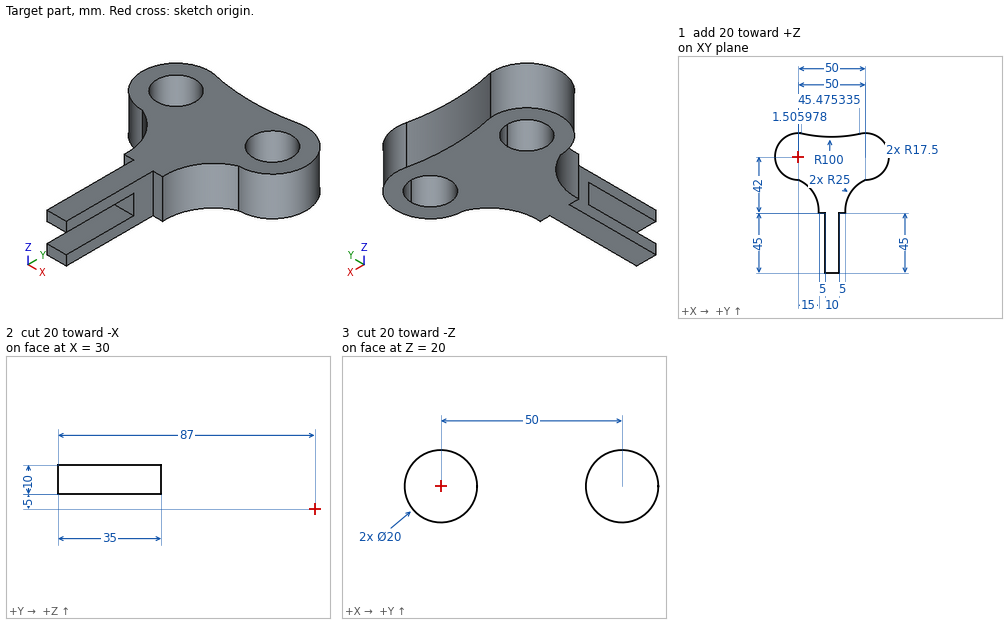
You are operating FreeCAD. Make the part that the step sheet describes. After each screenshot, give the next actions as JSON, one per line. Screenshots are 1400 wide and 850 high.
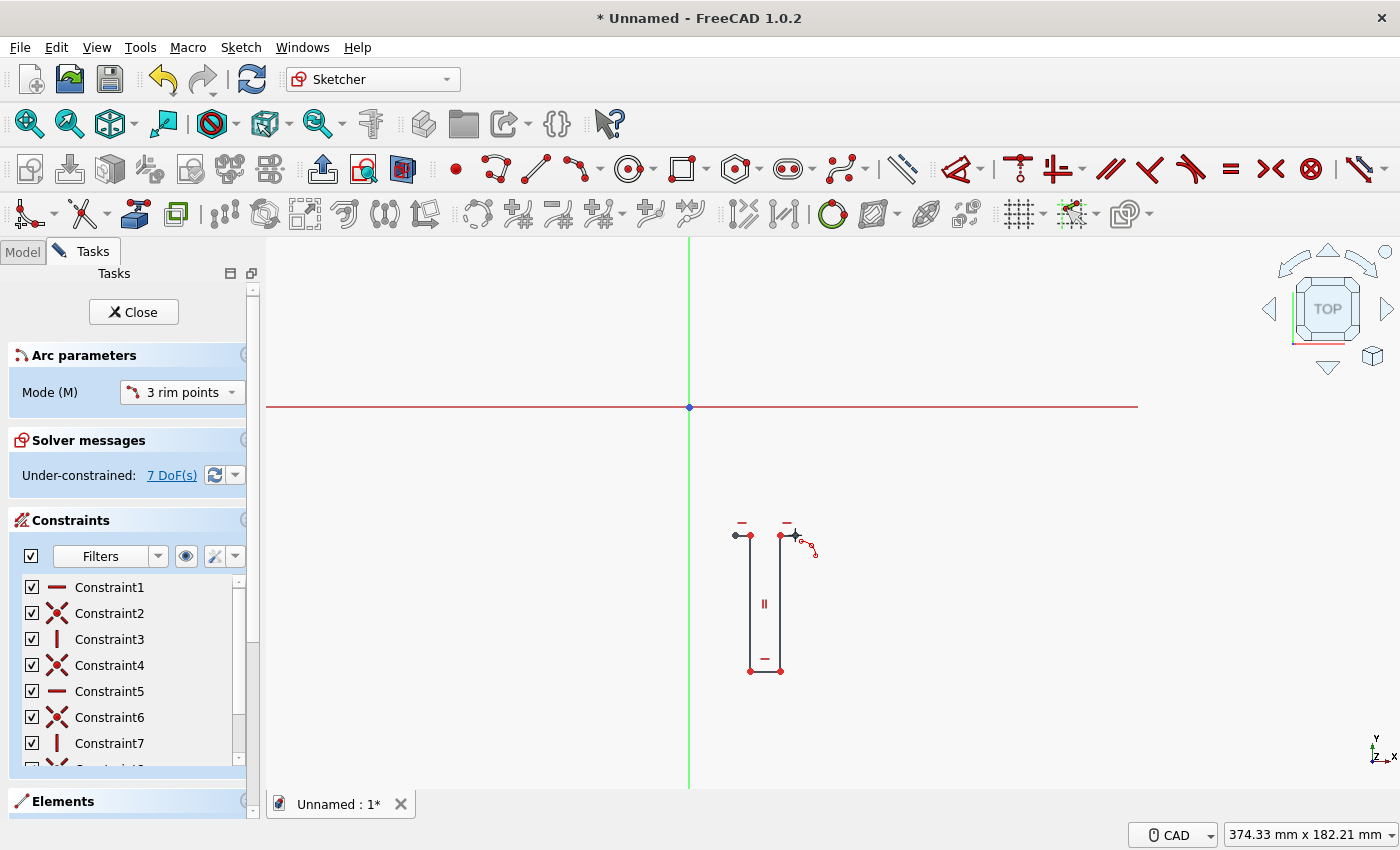
{"action": "scroll", "coordinate": [795, 535], "scroll_direction": "up", "scroll_amount": 4}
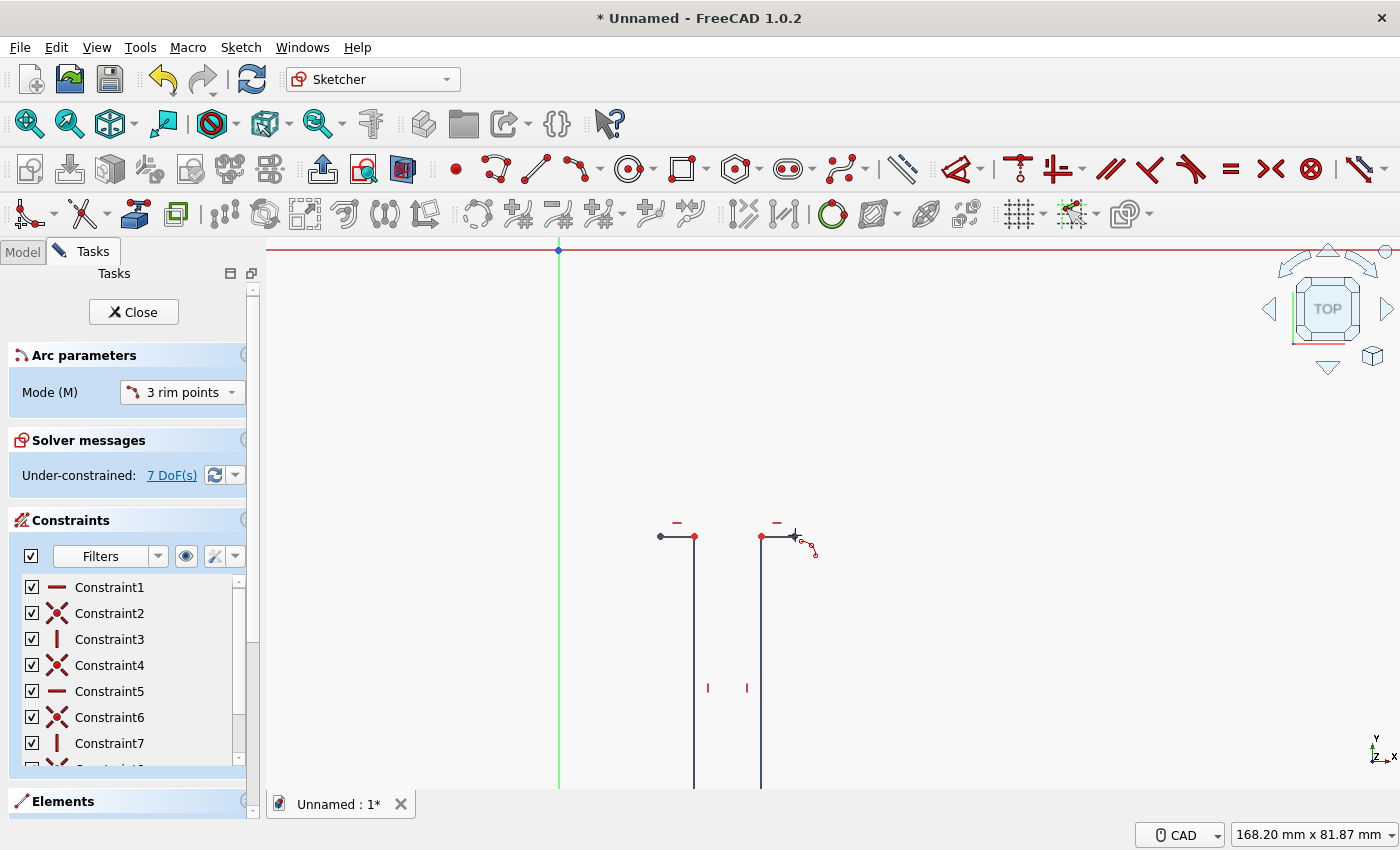
{"action": "left_click", "coordinate": [794, 537]}
{"action": "left_click", "coordinate": [896, 368]}
{"action": "left_click", "coordinate": [819, 435]}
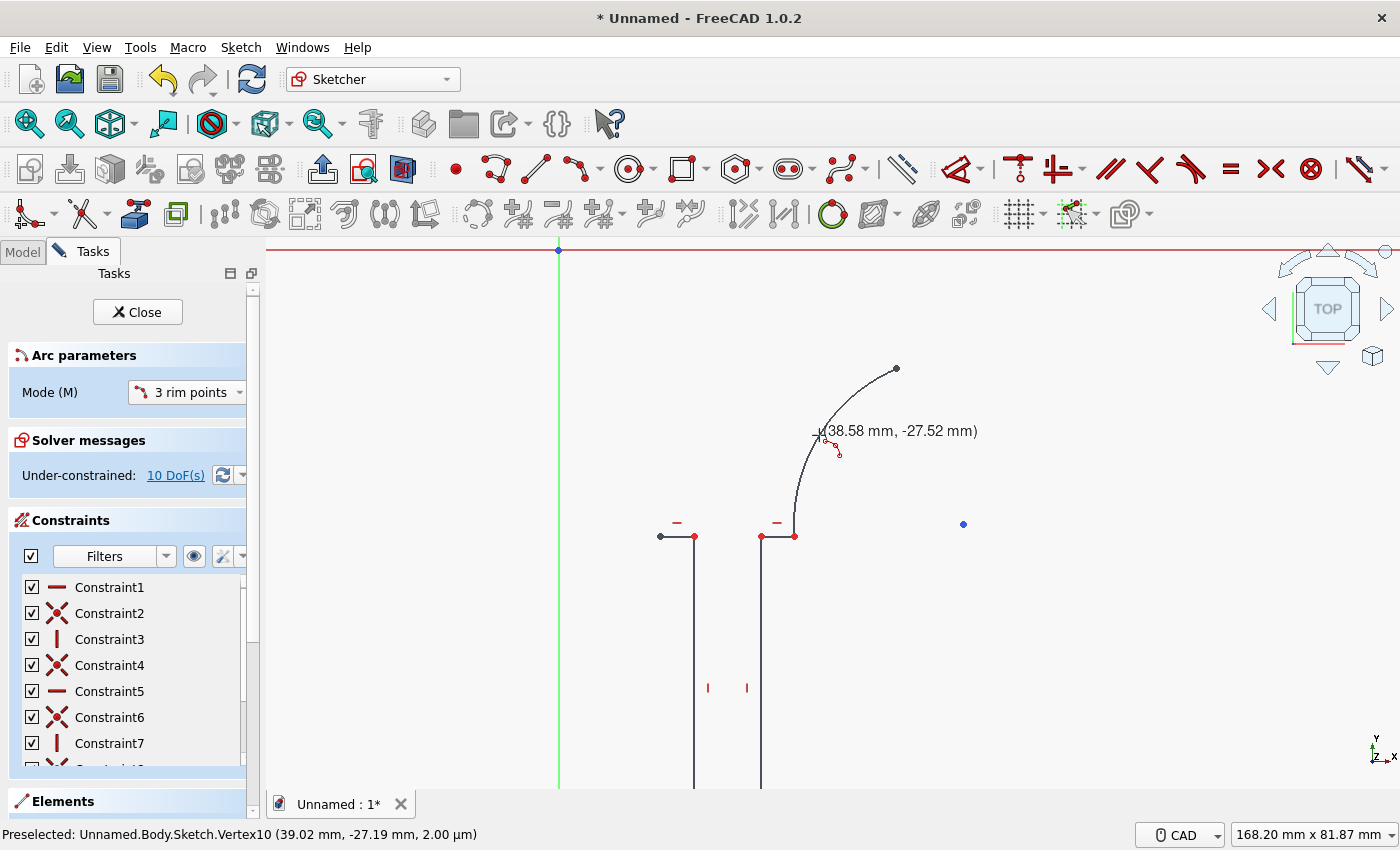
{"action": "left_click", "coordinate": [896, 369]}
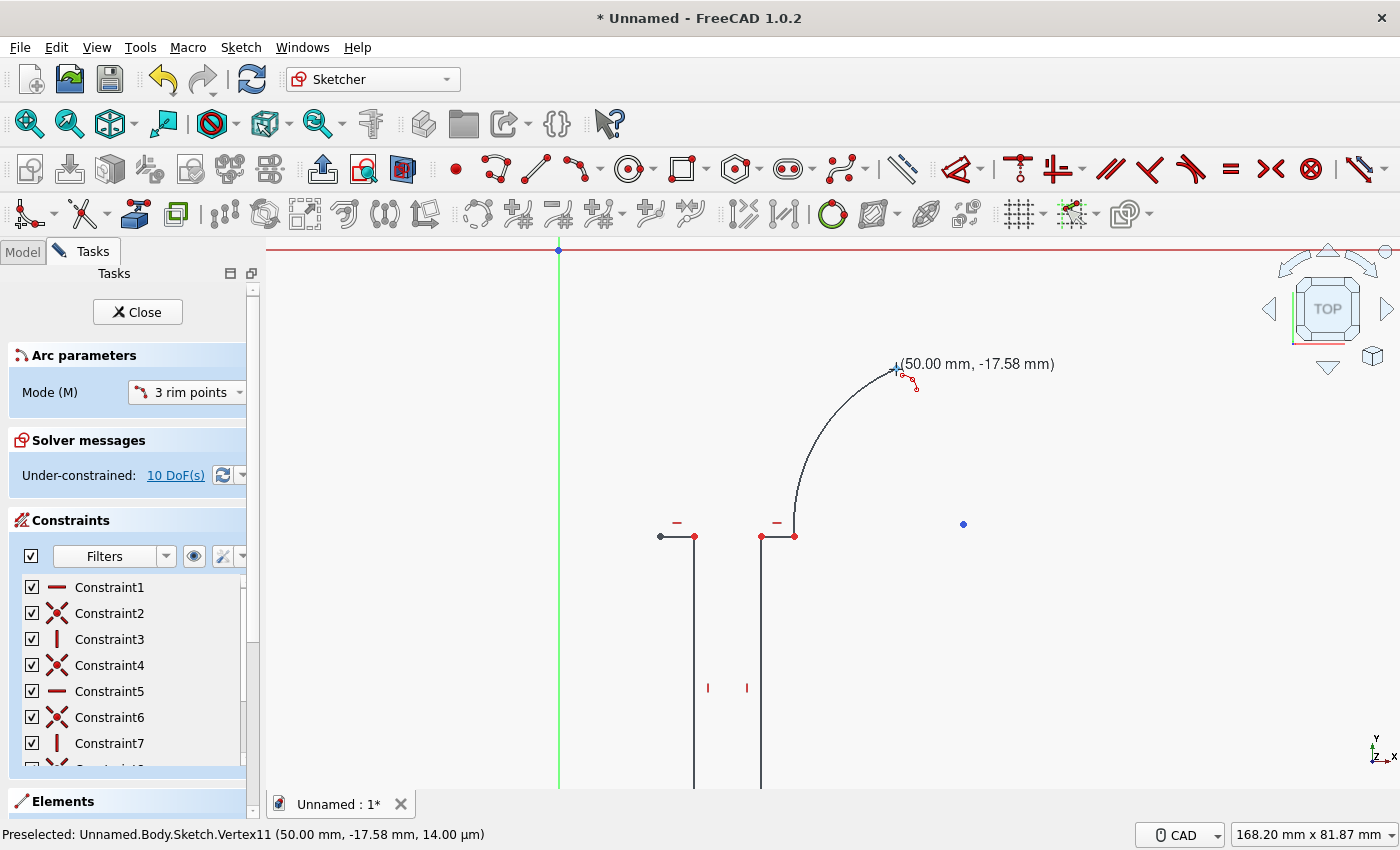
{"action": "scroll", "coordinate": [810, 547], "scroll_direction": "down", "scroll_amount": 3}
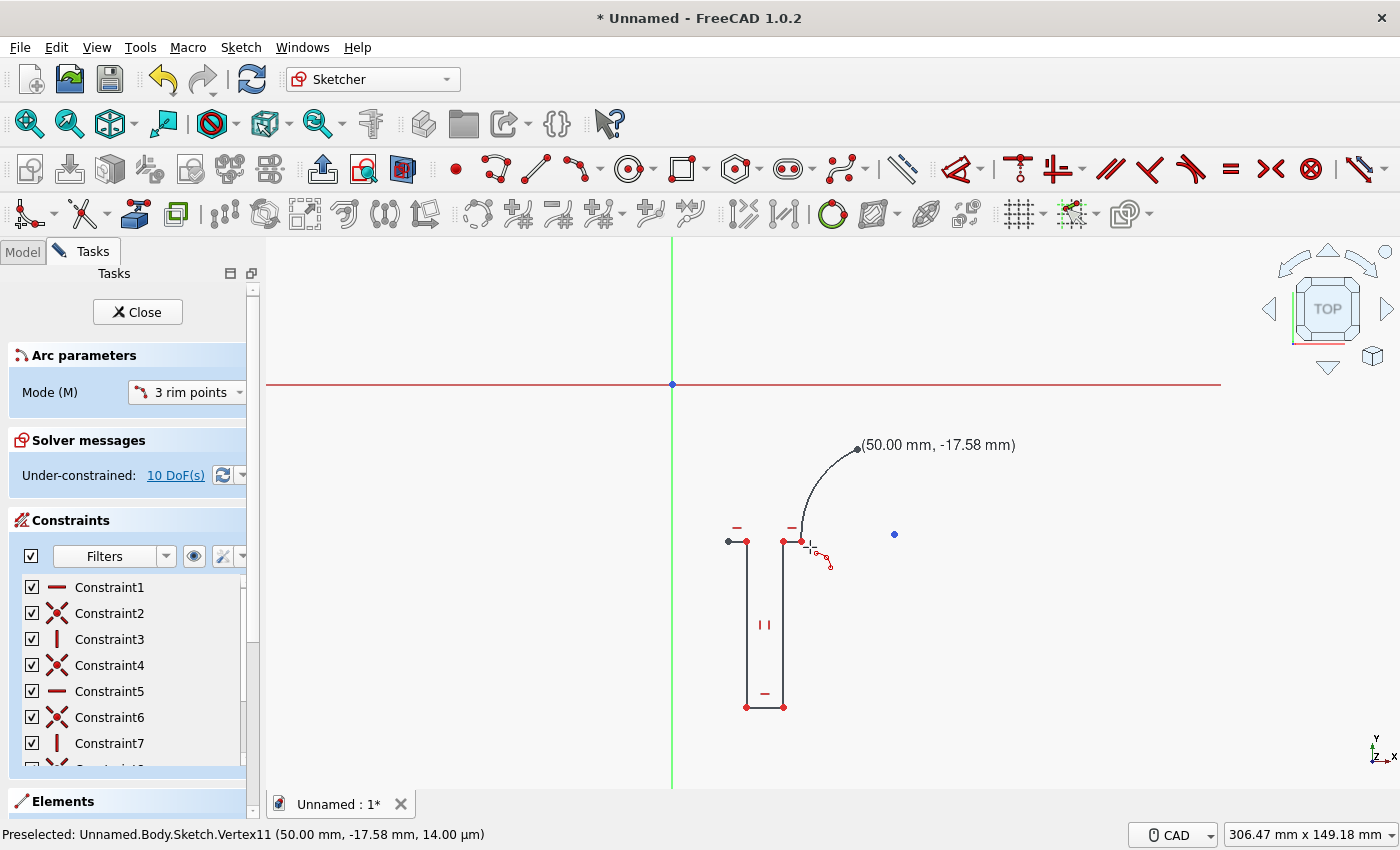
{"action": "left_click", "coordinate": [841, 322]}
{"action": "left_click", "coordinate": [915, 355]}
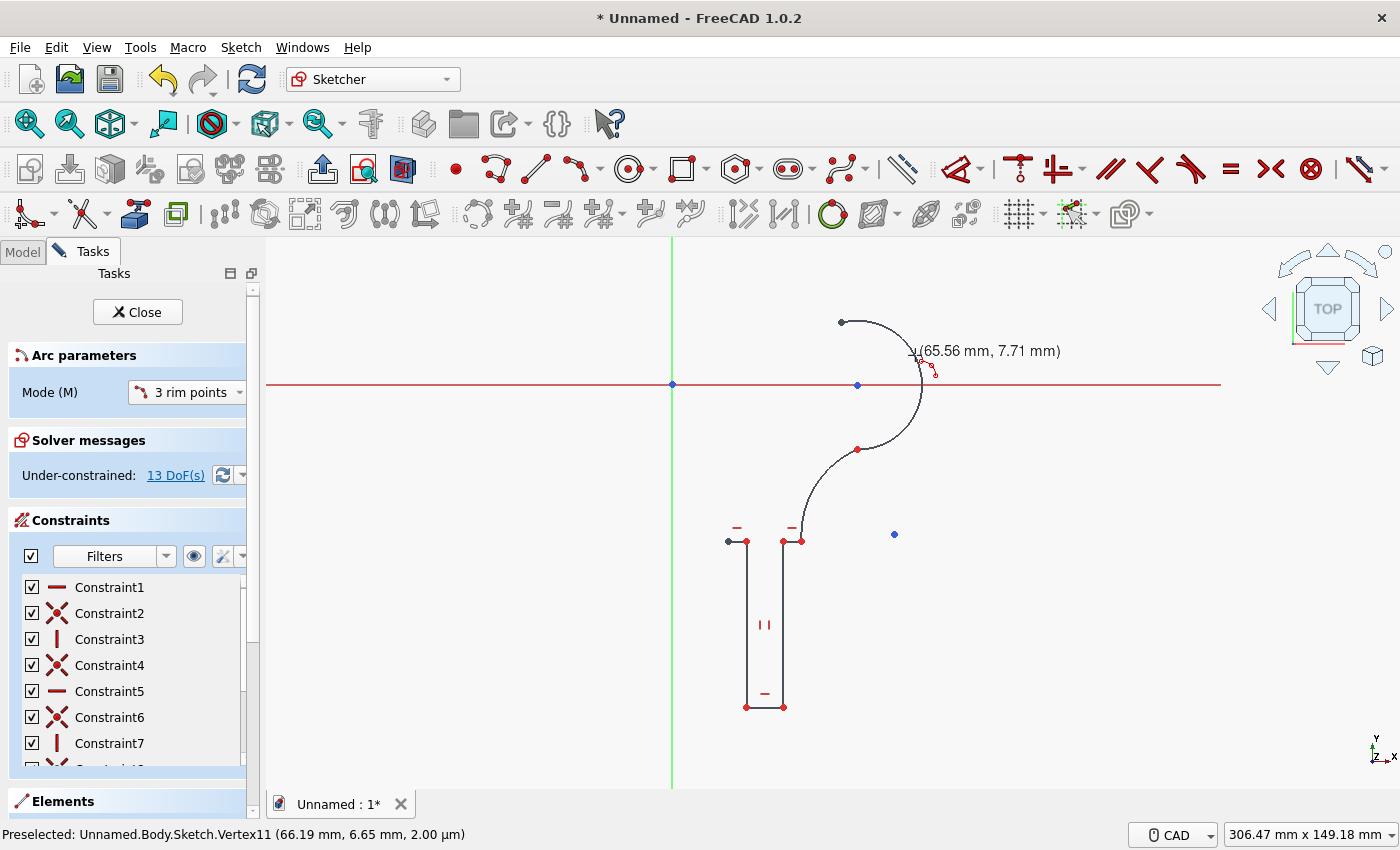
{"action": "left_click", "coordinate": [841, 323]}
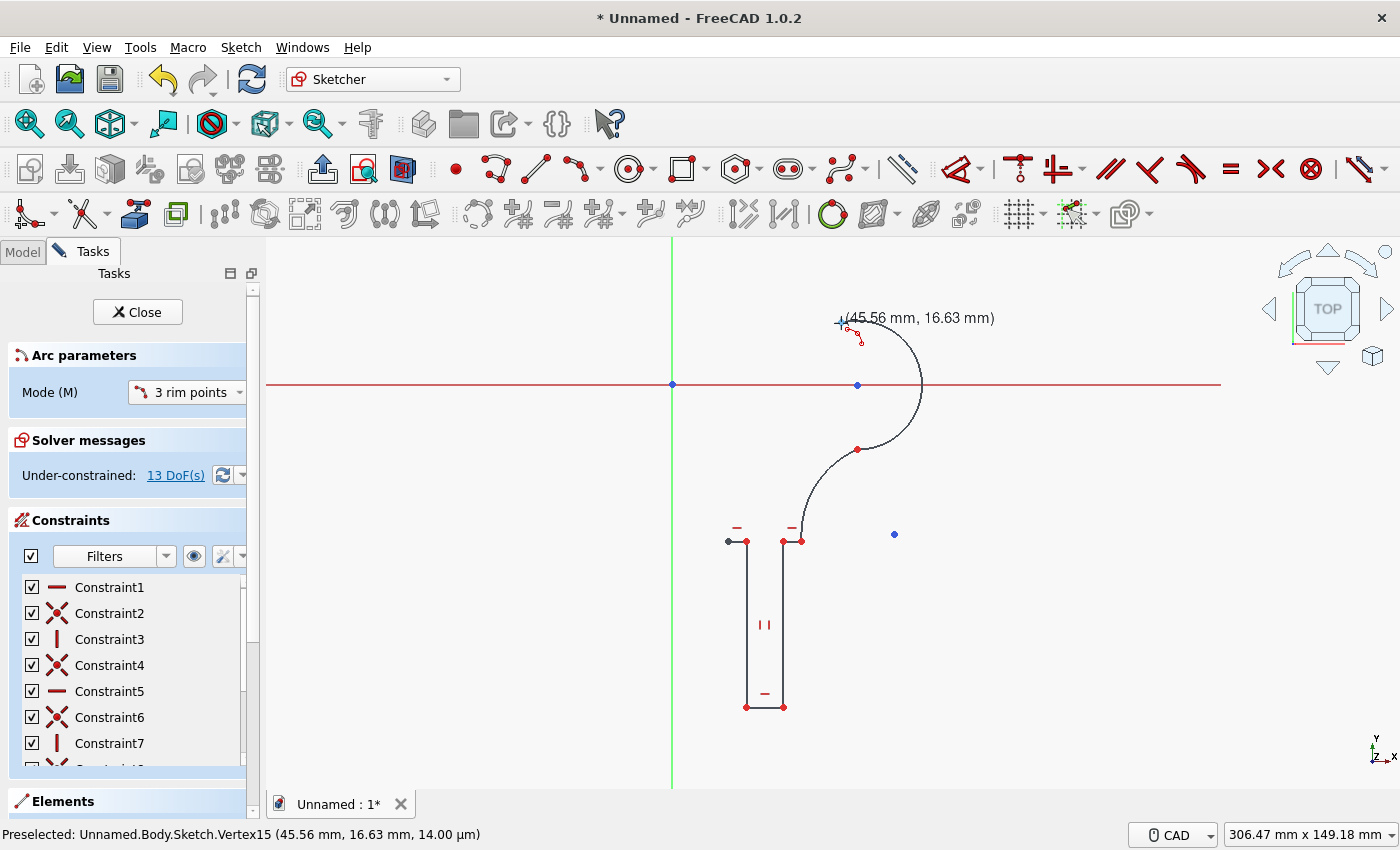
{"action": "scroll", "coordinate": [678, 320], "scroll_direction": "up", "scroll_amount": 6}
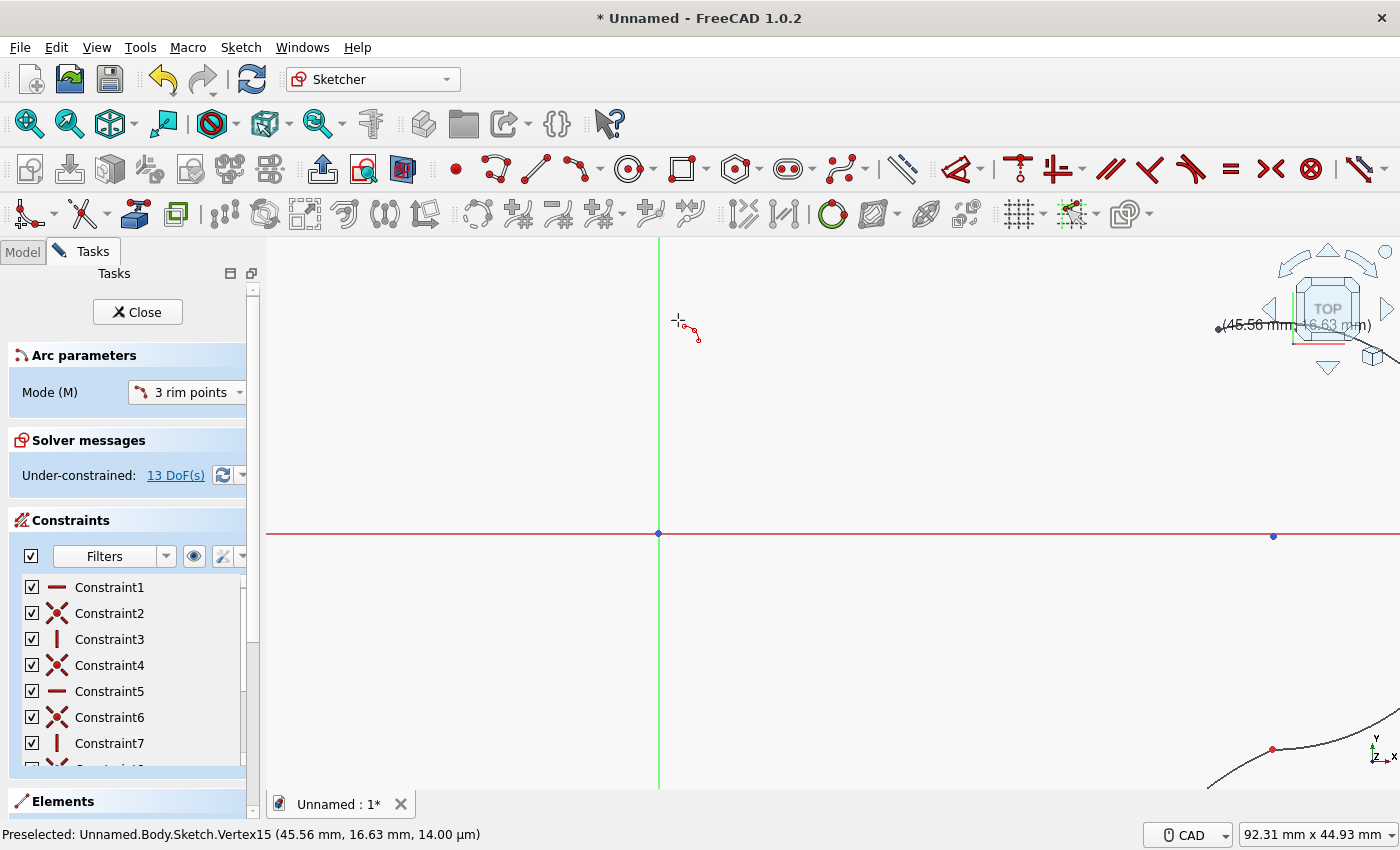
{"action": "left_click", "coordinate": [677, 320]}
{"action": "left_click", "coordinate": [947, 353]}